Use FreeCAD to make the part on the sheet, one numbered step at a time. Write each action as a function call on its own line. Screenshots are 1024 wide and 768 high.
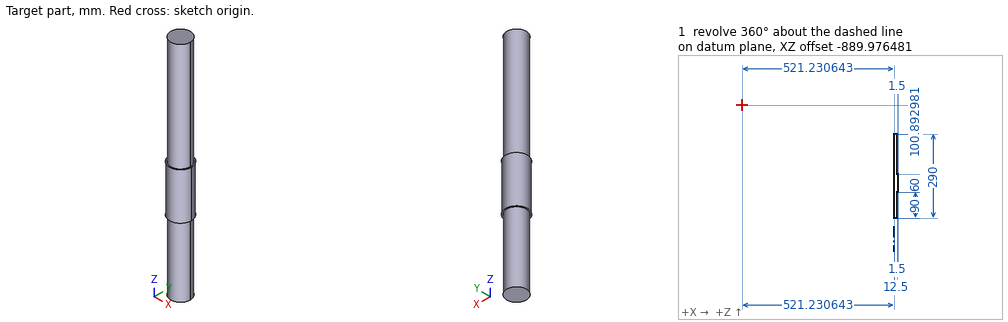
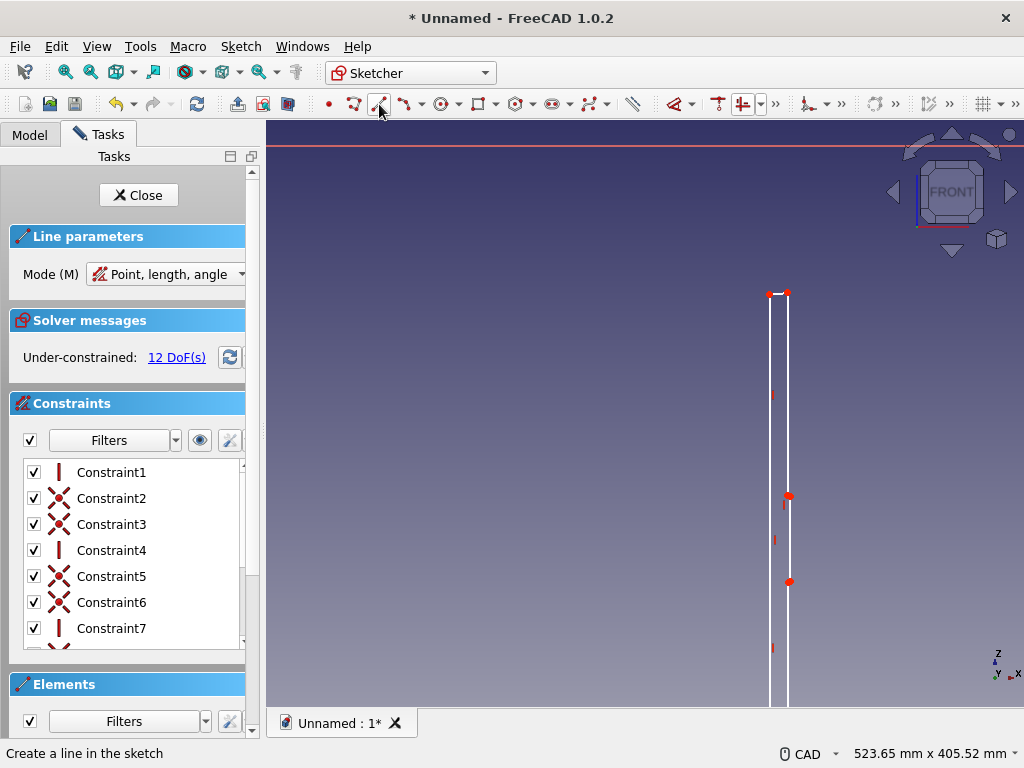
scroll(788, 292, down, 3)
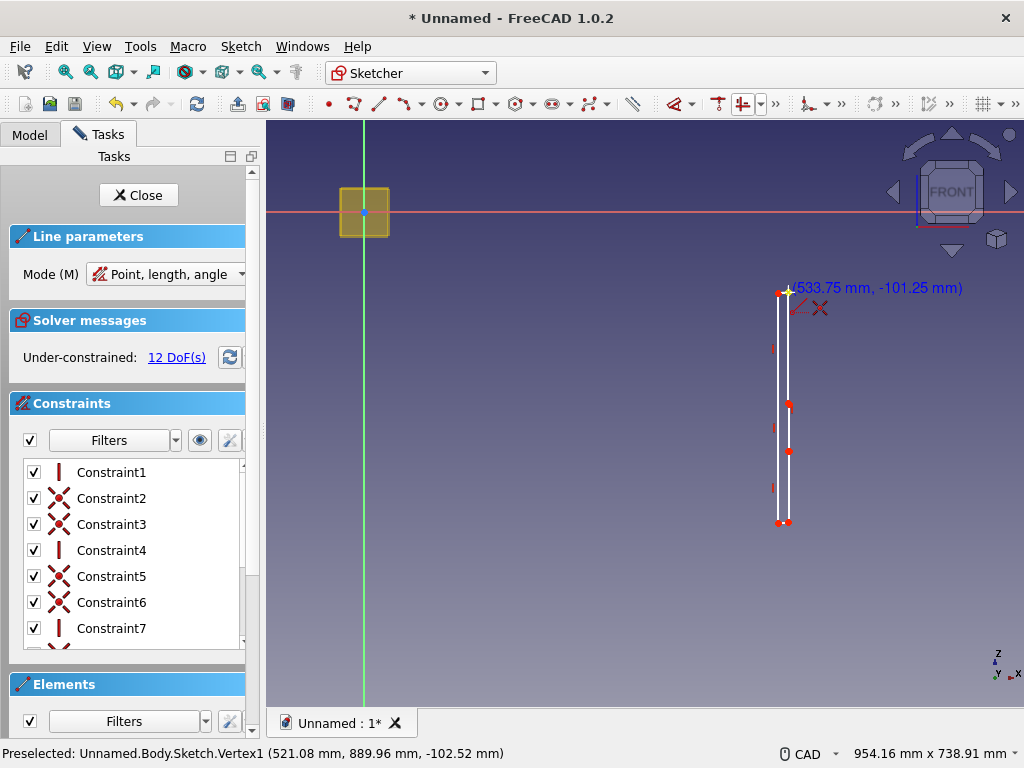
click(778, 546)
click(778, 615)
key(Escape)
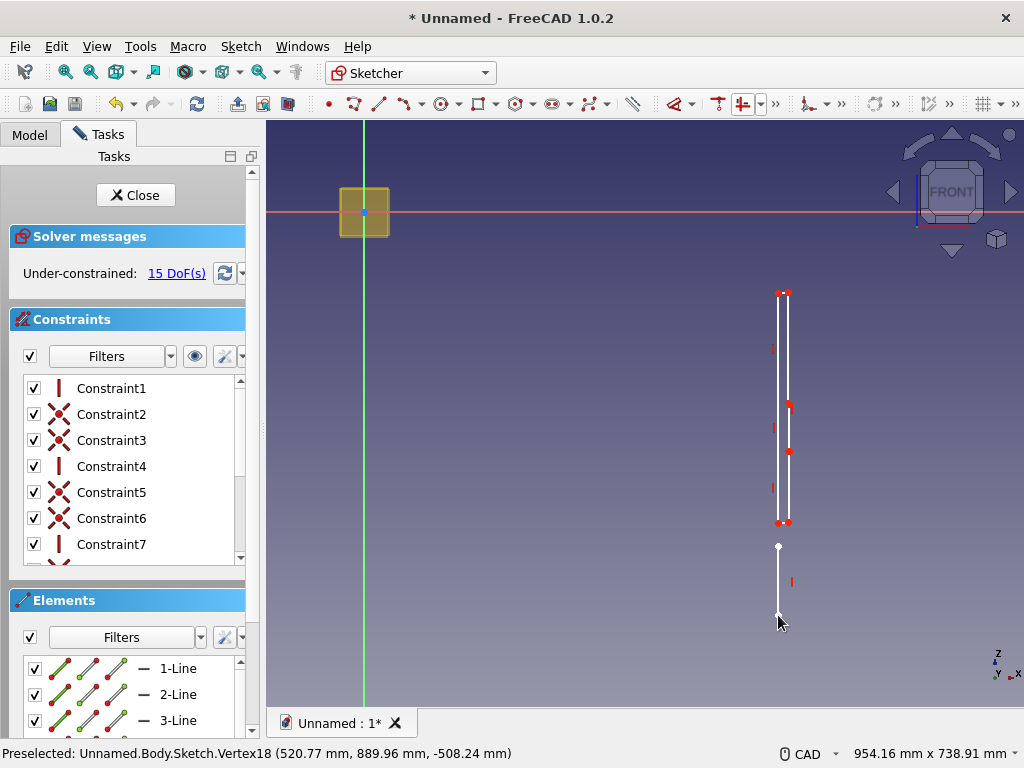
click(778, 568)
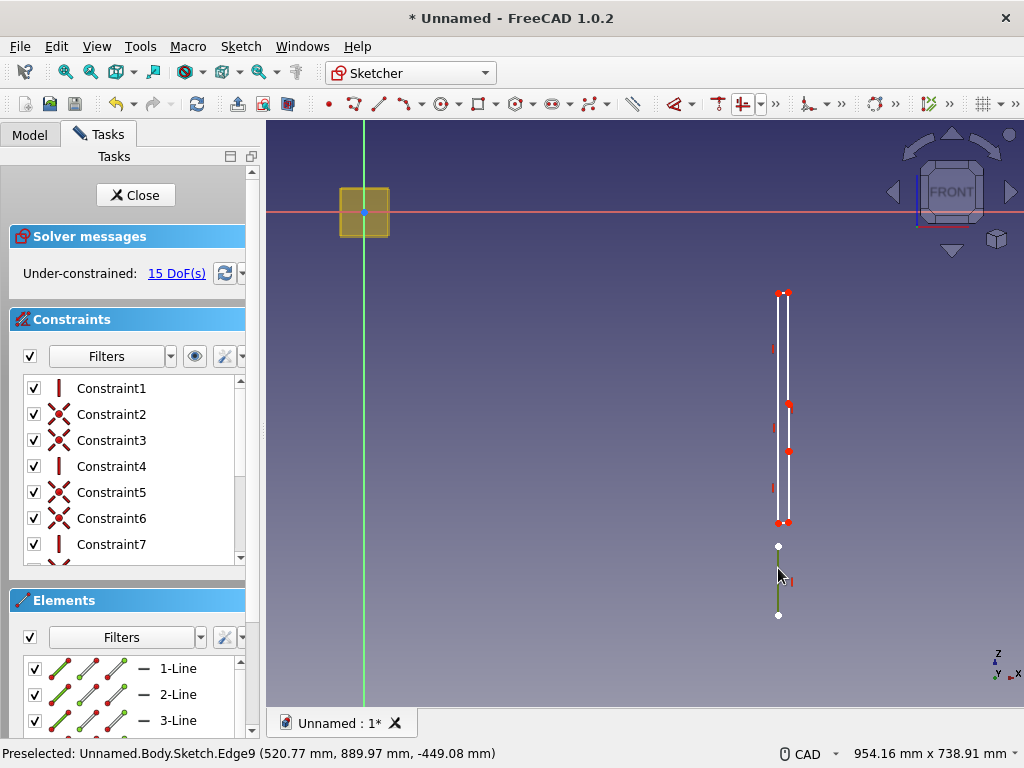
key(g)
key(n)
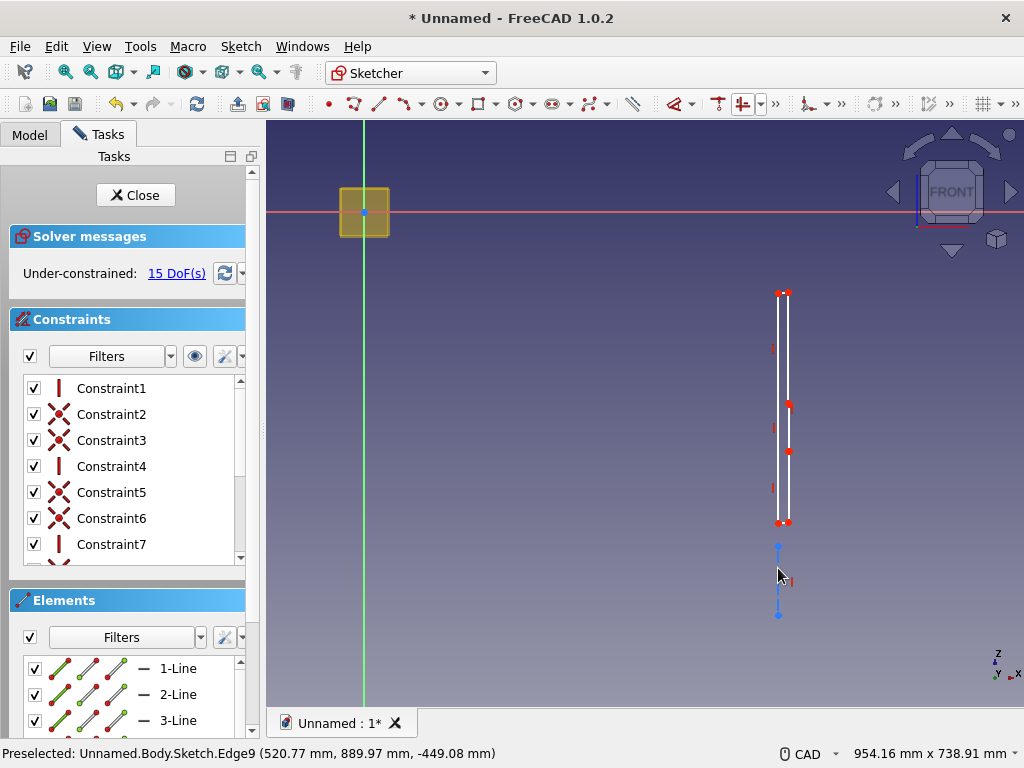
scroll(783, 523, up, 5)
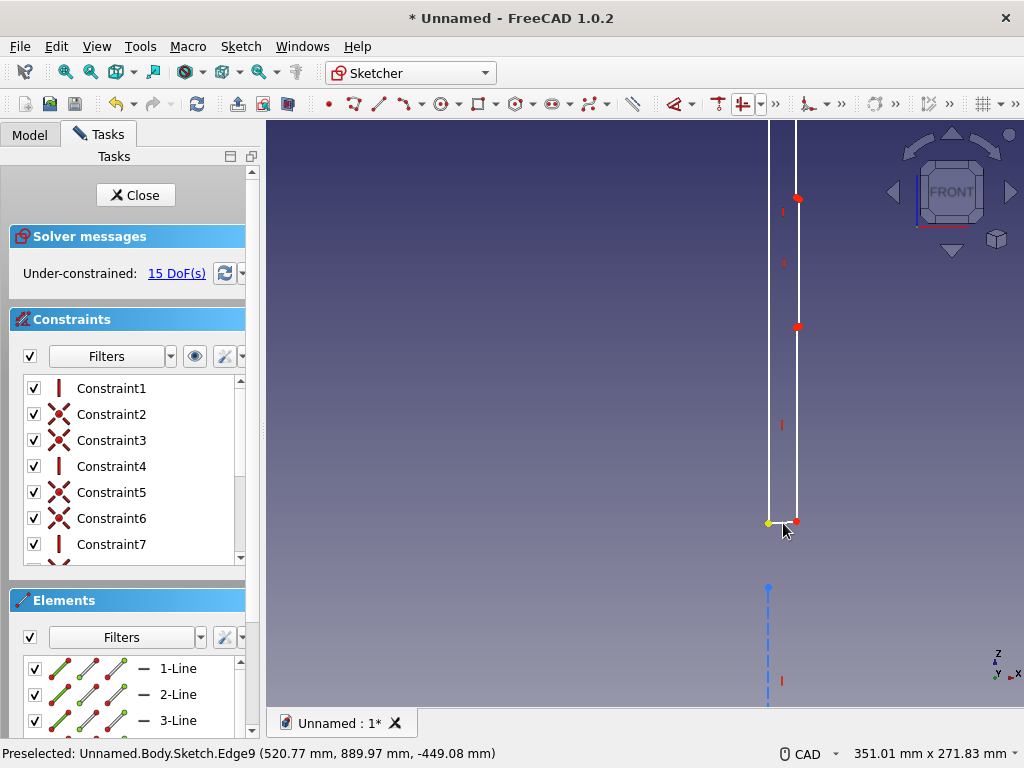
click(783, 523)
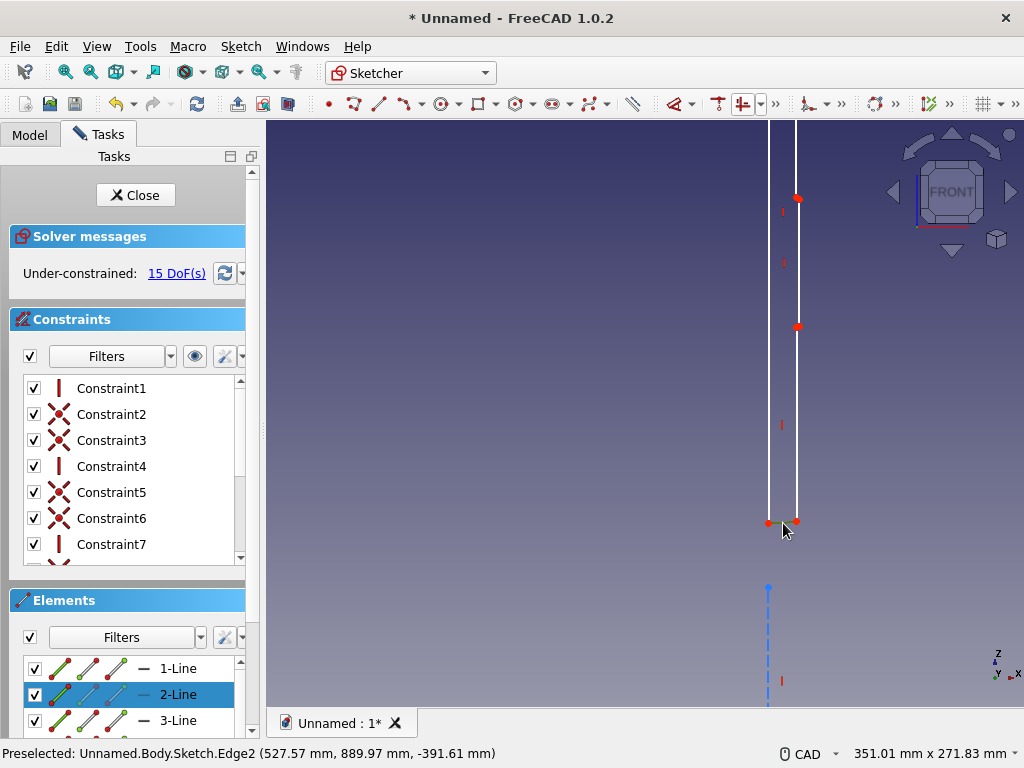
click(760, 104)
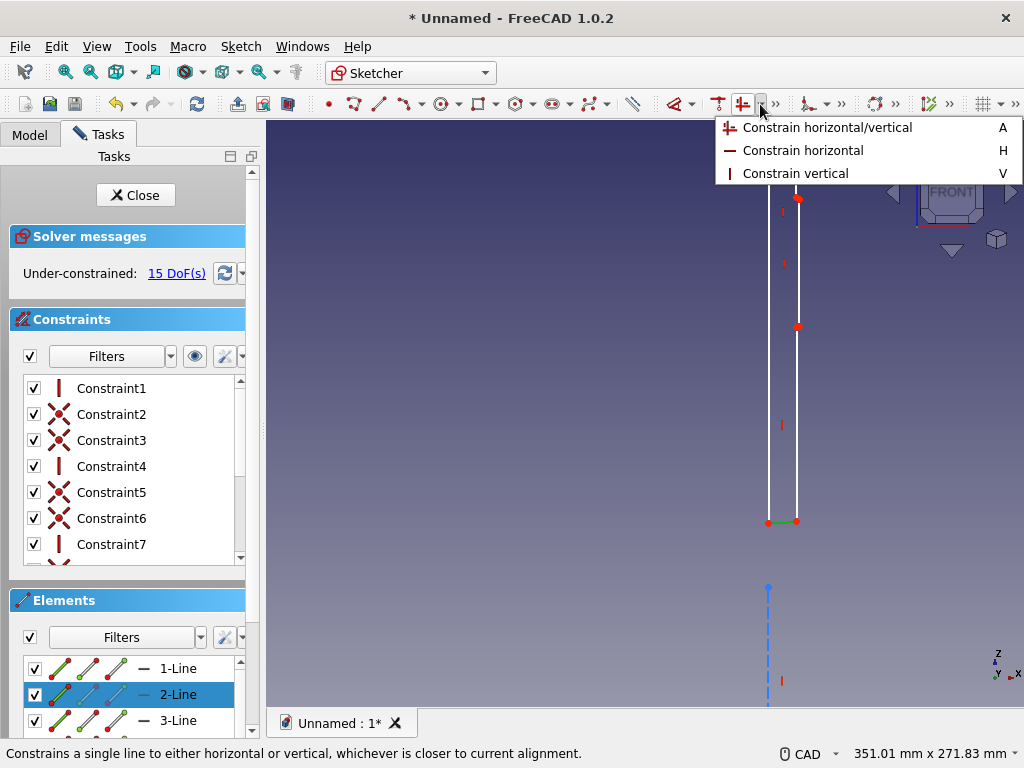
click(869, 150)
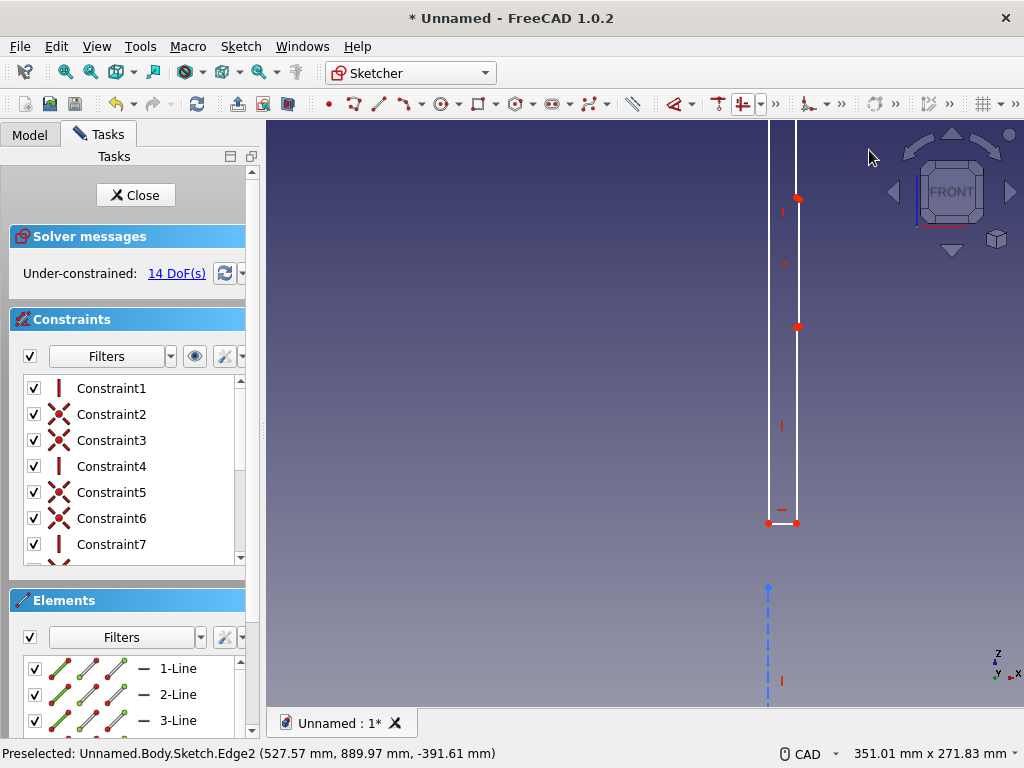
scroll(798, 327, up, 9)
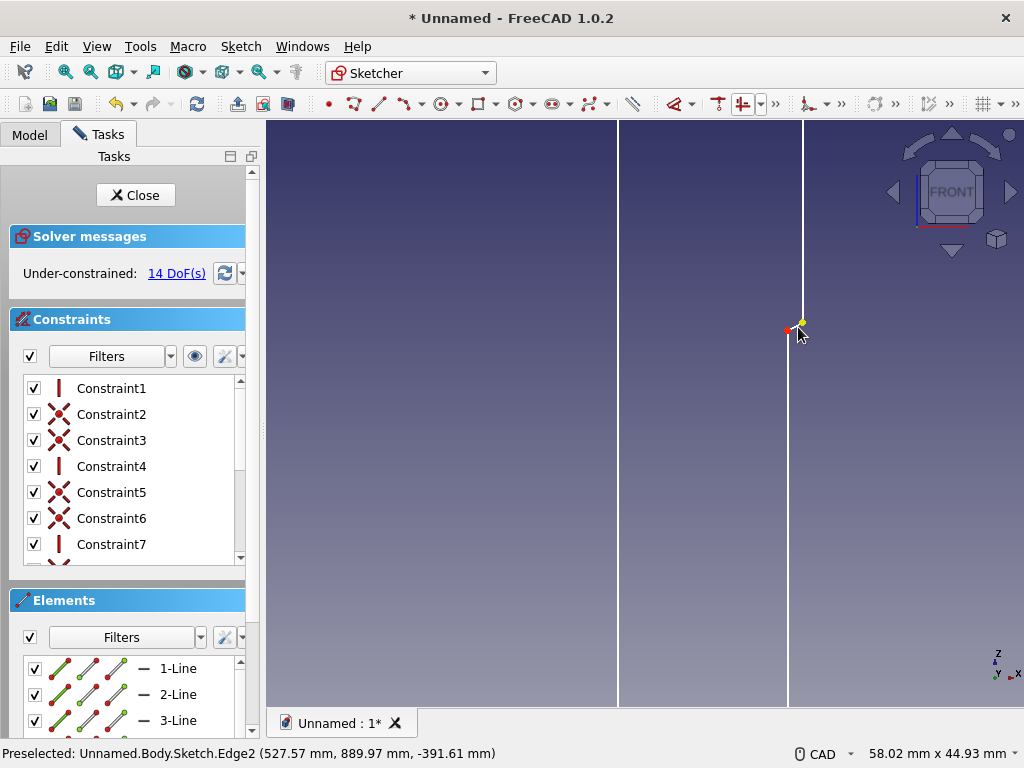
click(795, 327)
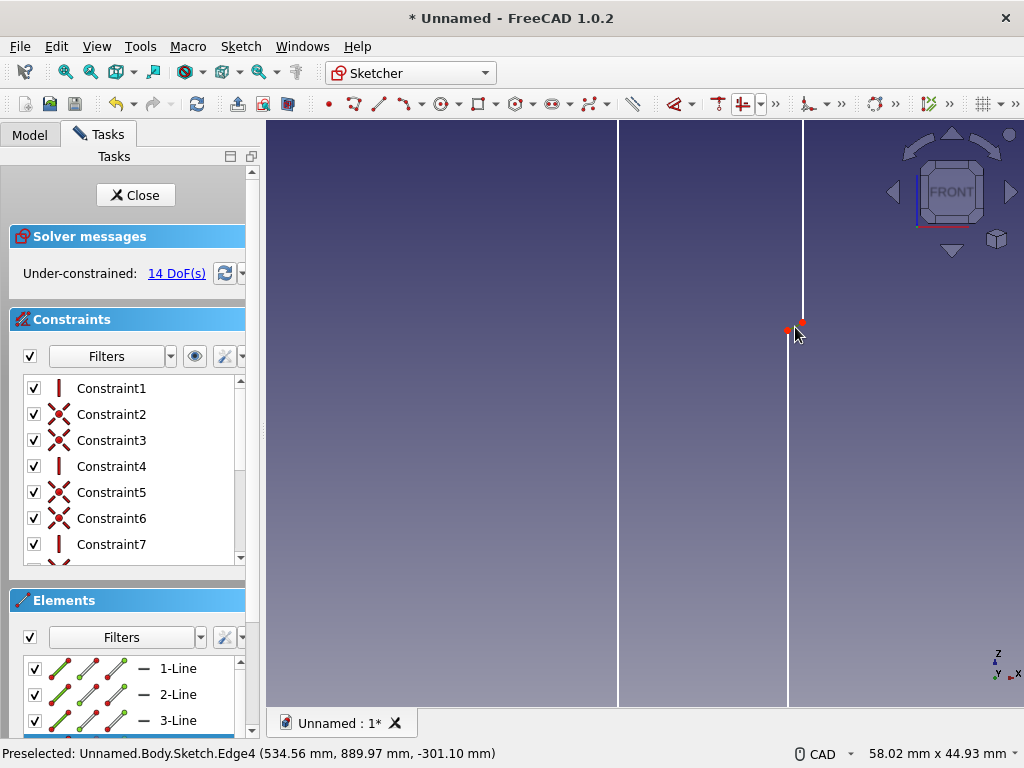
click(760, 104)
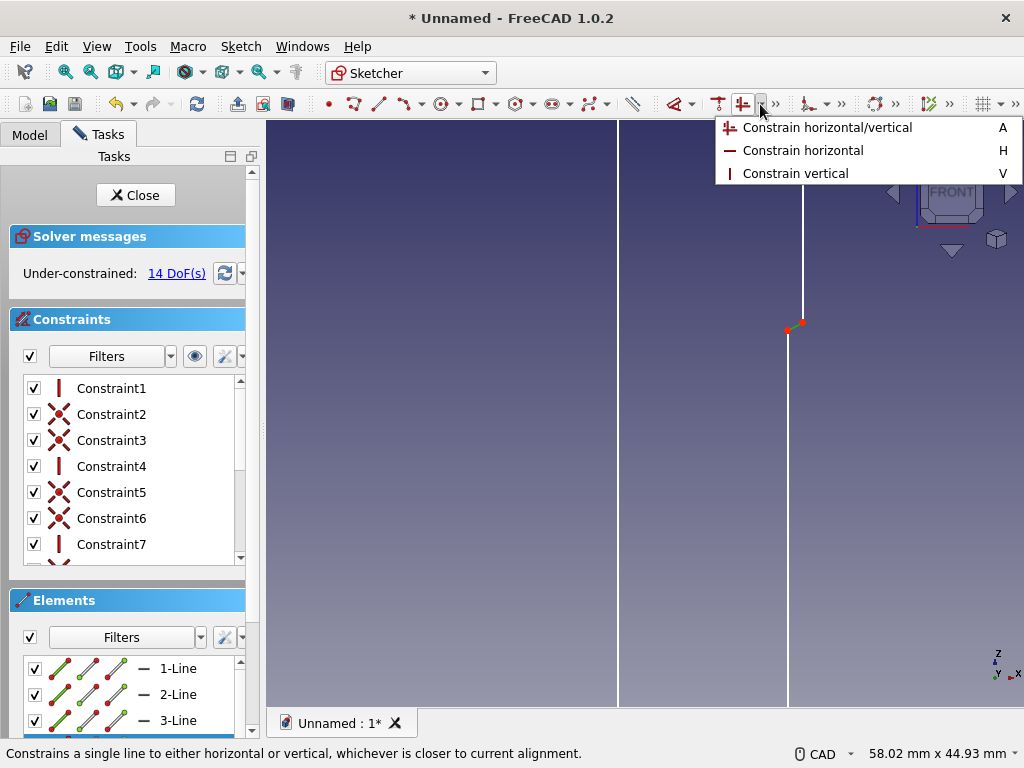
click(869, 150)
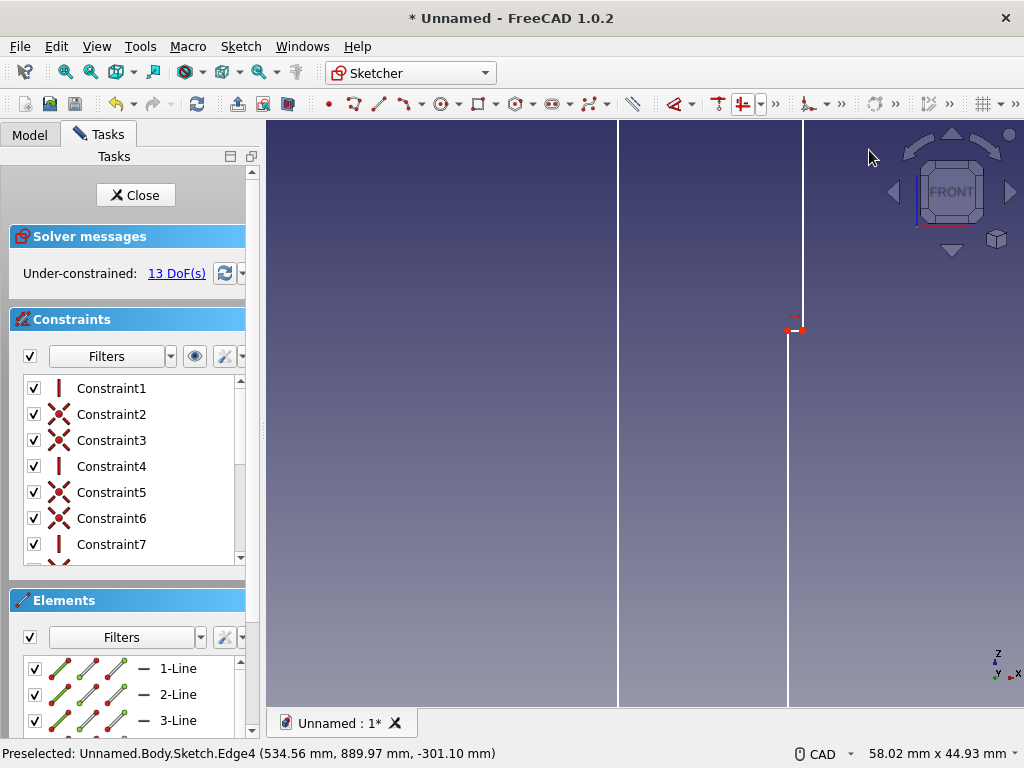
scroll(788, 459, down, 14)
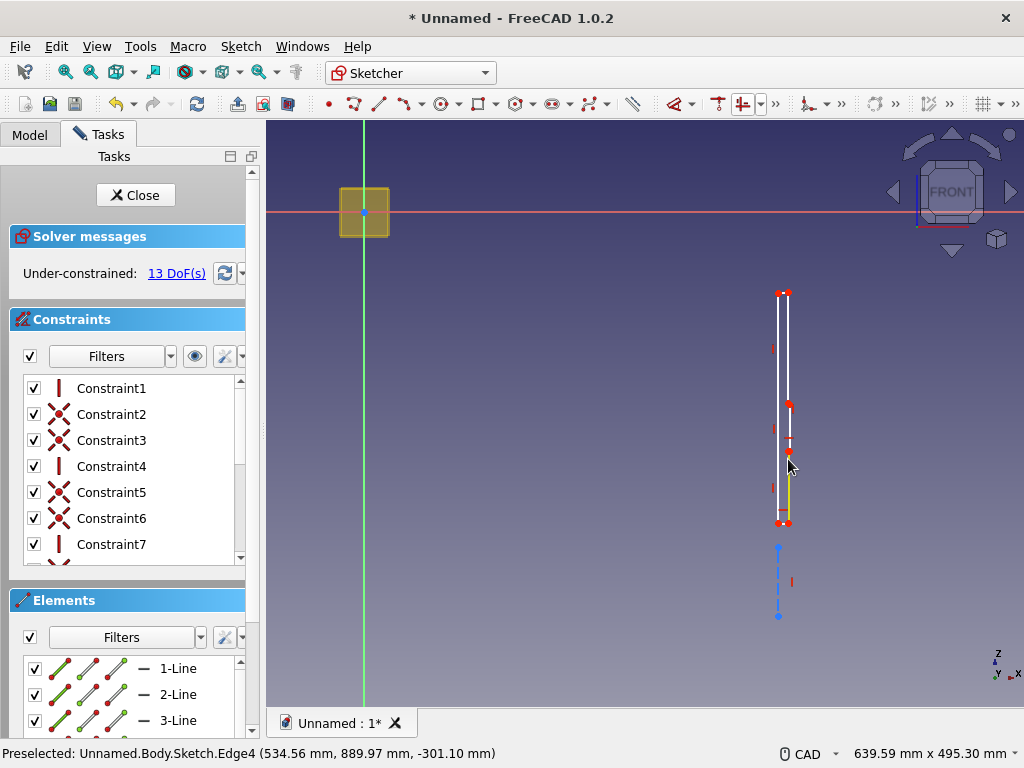
scroll(789, 404, up, 14)